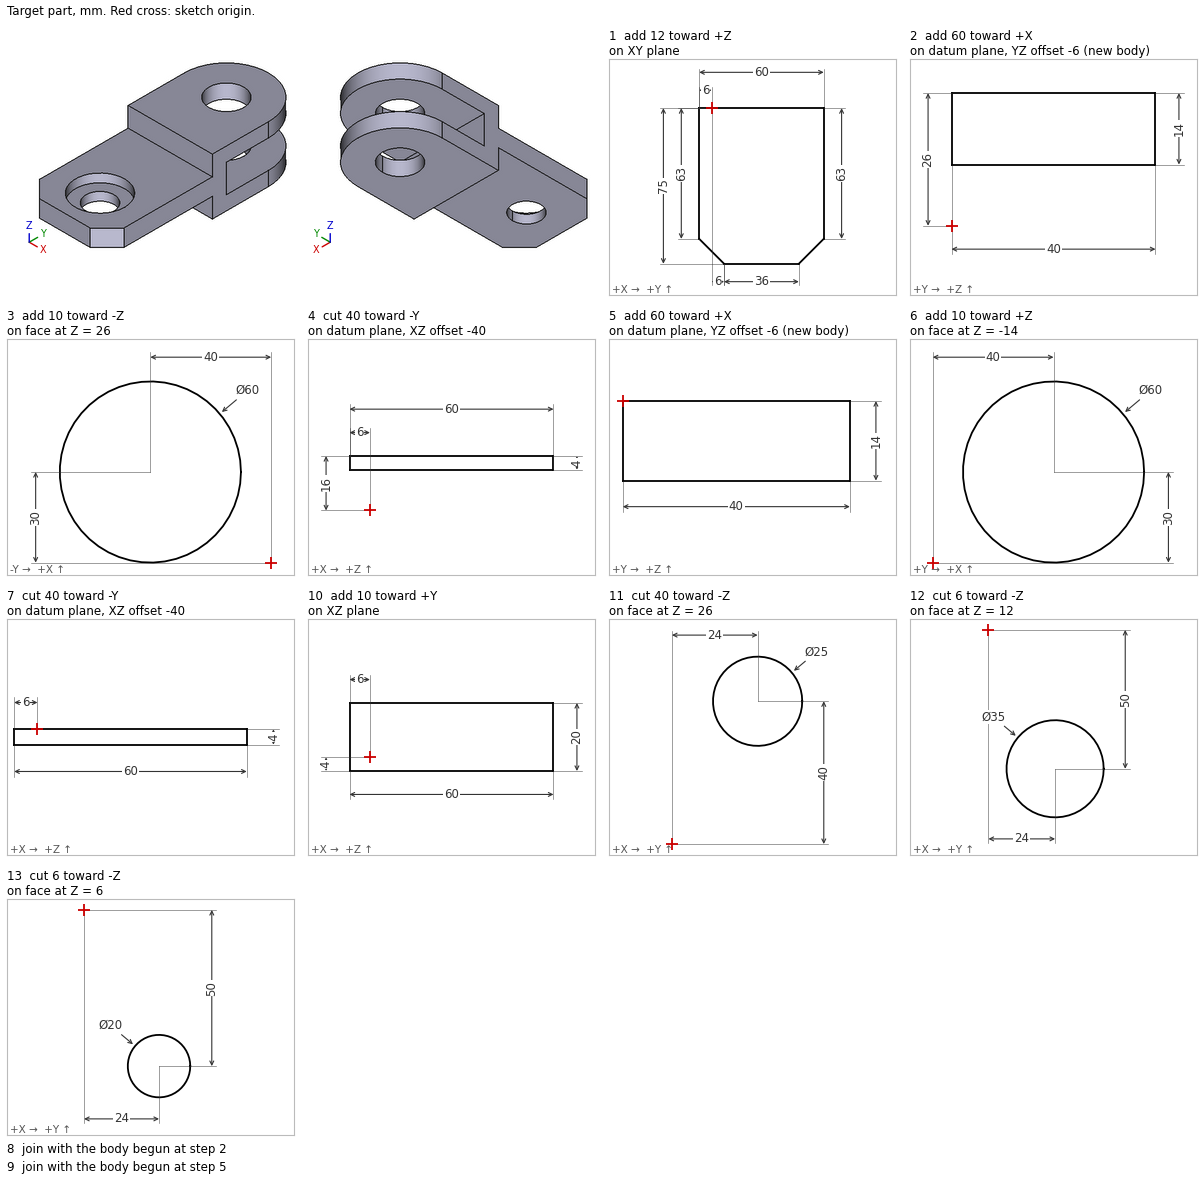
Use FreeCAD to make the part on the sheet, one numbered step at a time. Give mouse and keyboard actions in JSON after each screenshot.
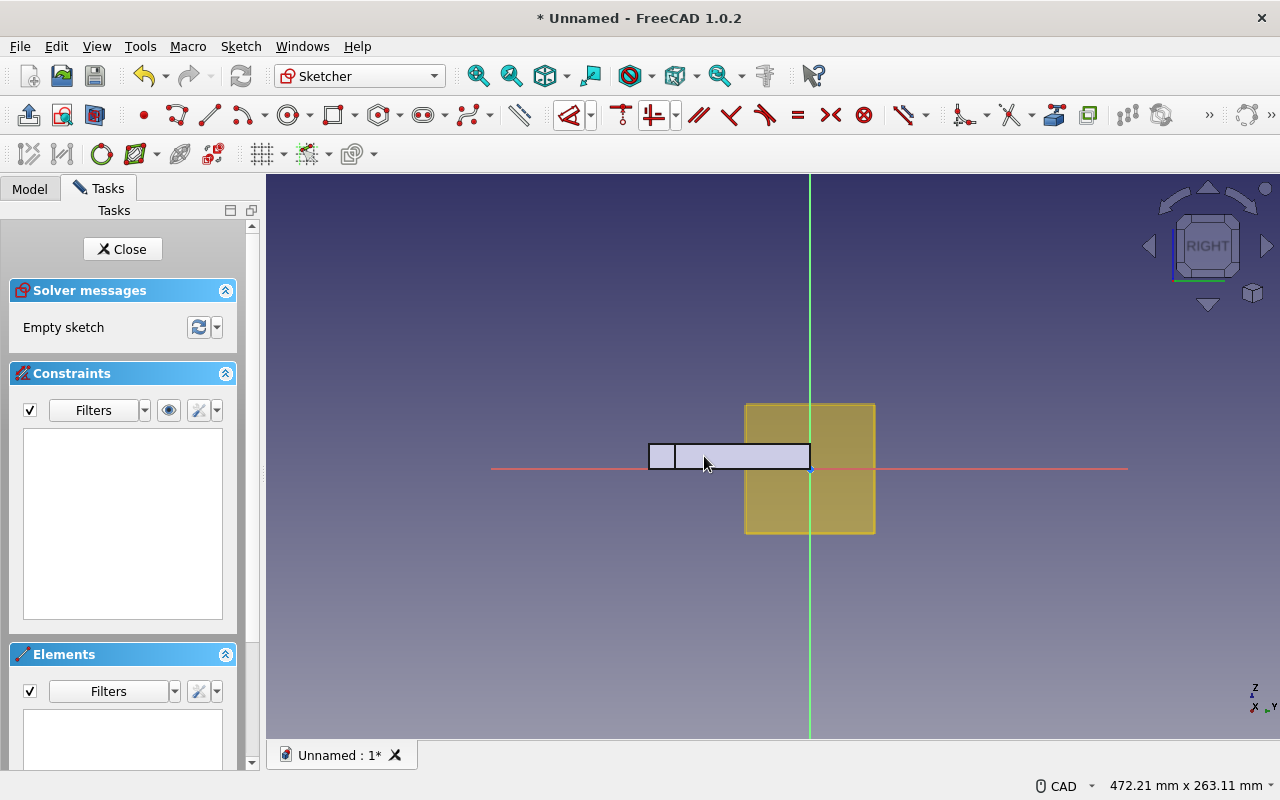
{"action": "scroll", "coordinate": [883, 438], "scroll_direction": "up", "scroll_amount": 9}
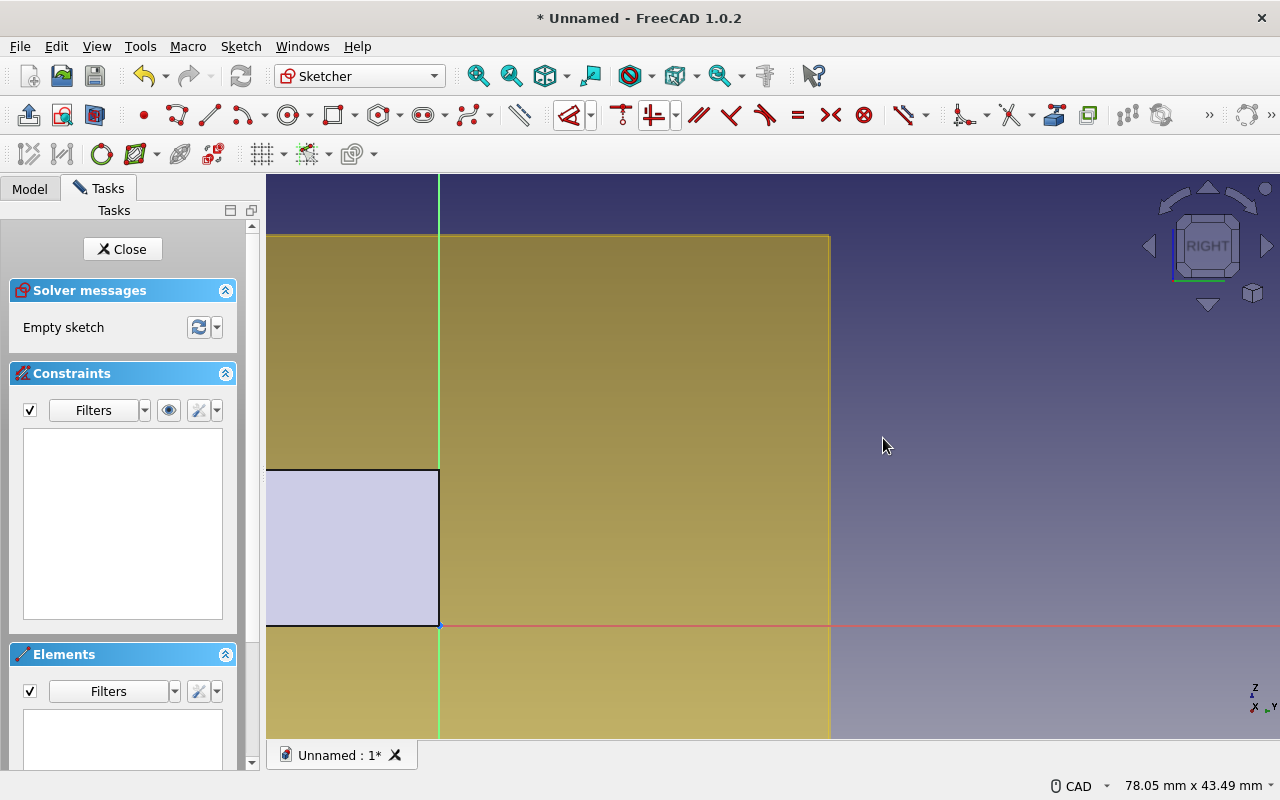
{"action": "left_click", "coordinate": [332, 116]}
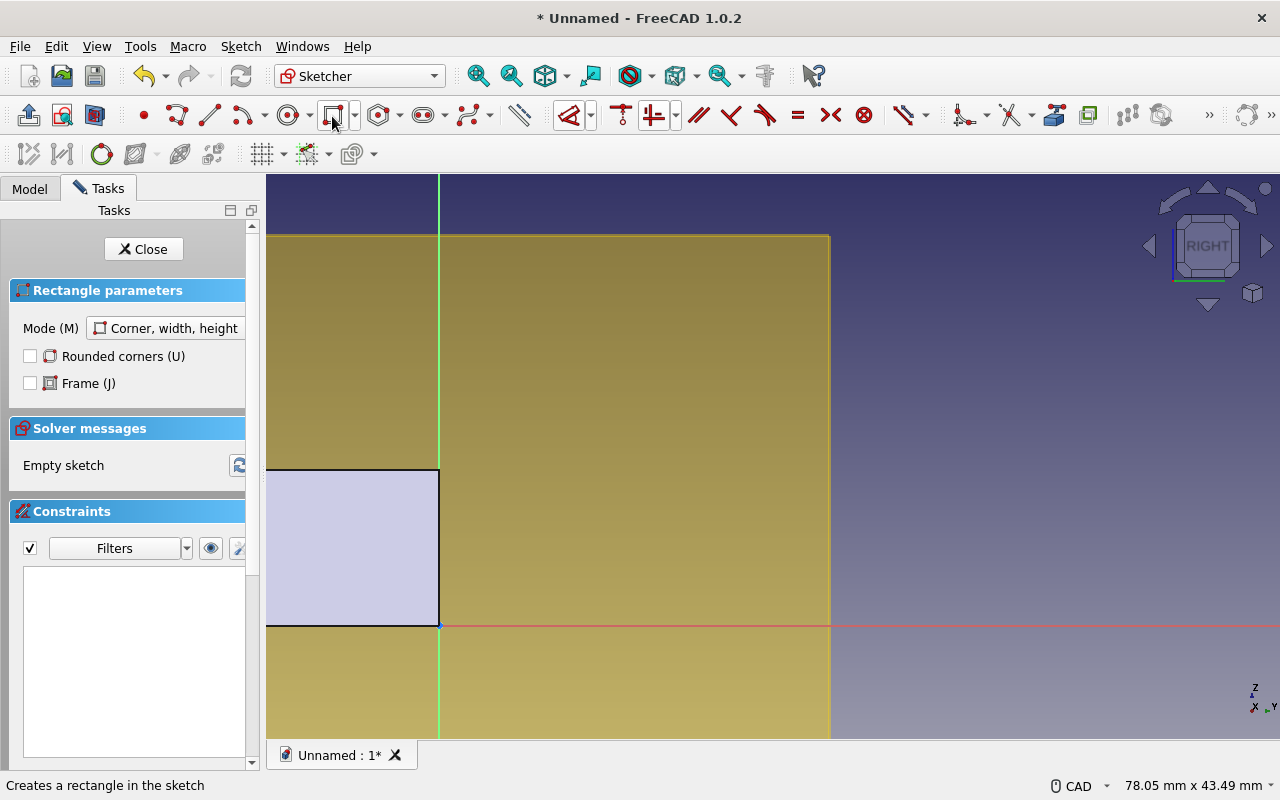
{"action": "left_click", "coordinate": [439, 288]}
{"action": "mouse_move", "coordinate": [959, 470]}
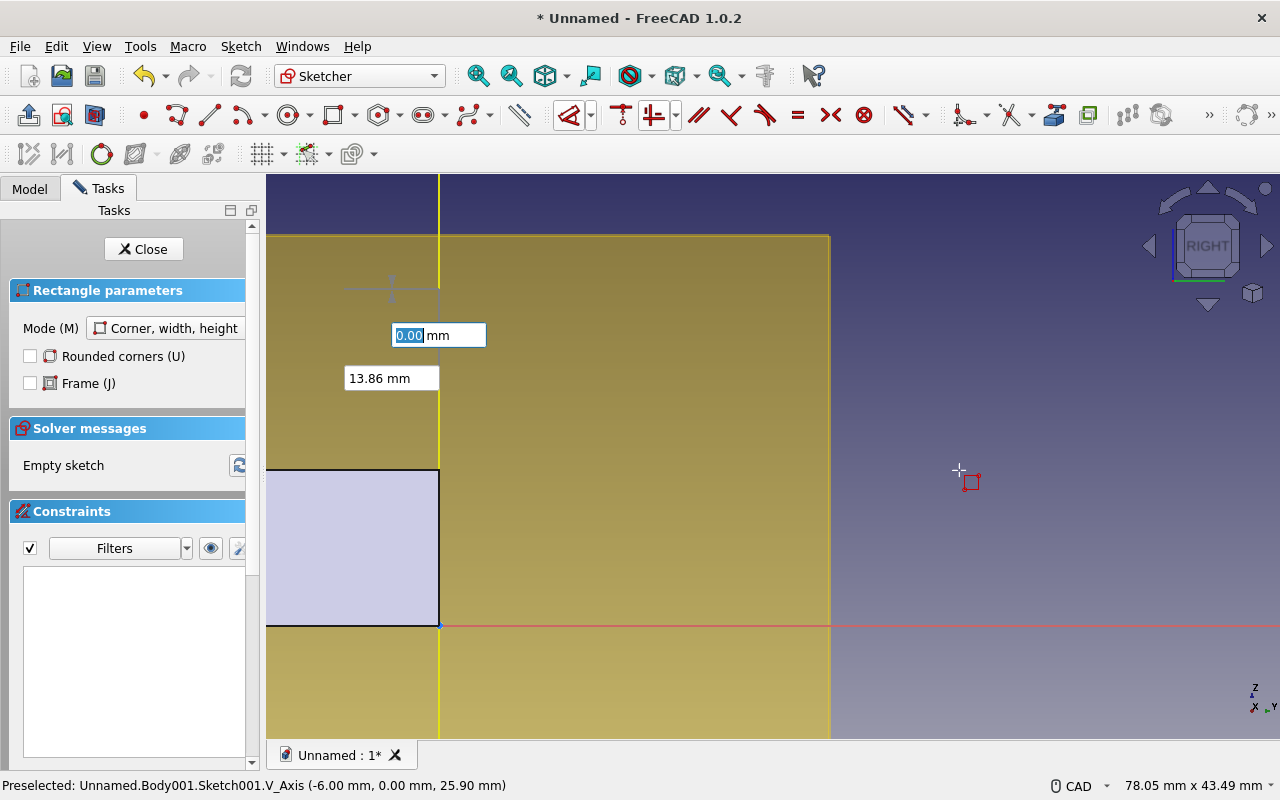
{"action": "type", "text": "40"}
{"action": "key", "text": "Tab"}
{"action": "type", "text": "14"}
{"action": "key", "text": "Return"}
{"action": "key", "text": "Escape"}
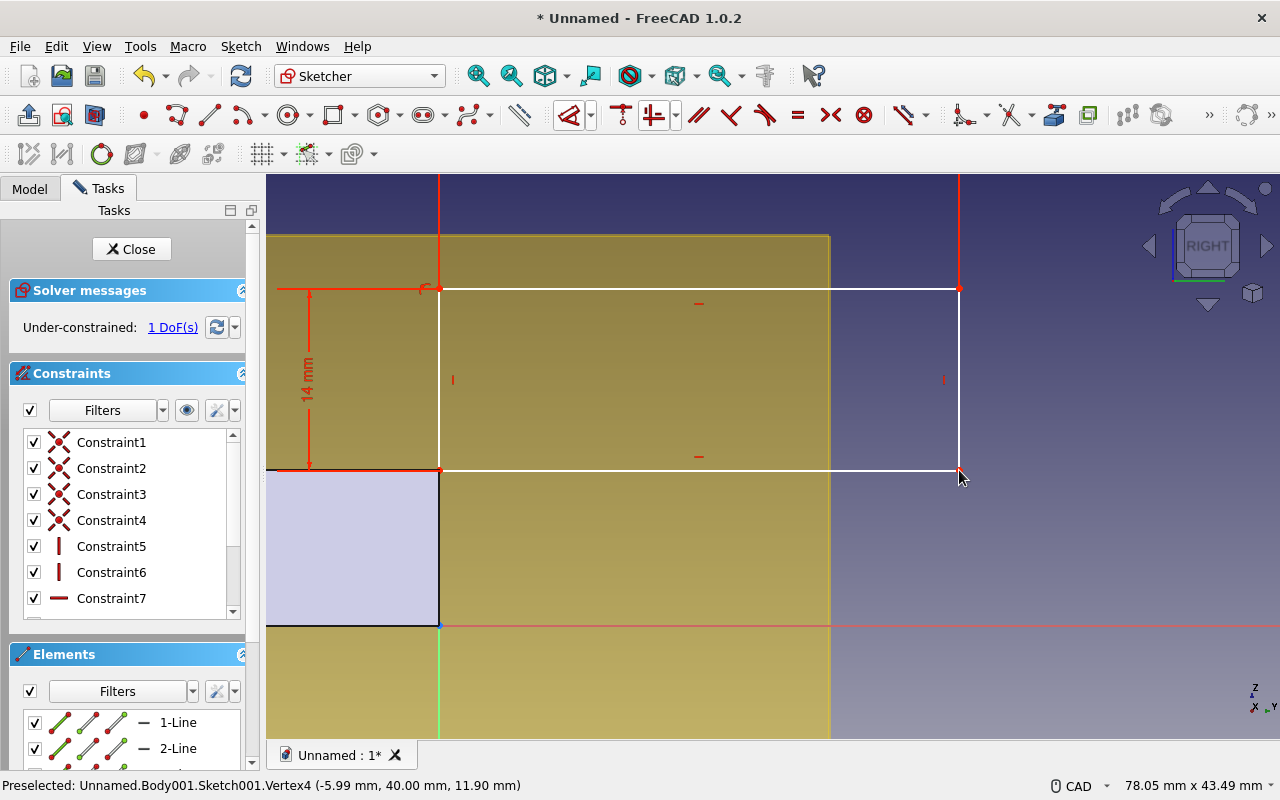
{"action": "left_click", "coordinate": [439, 289]}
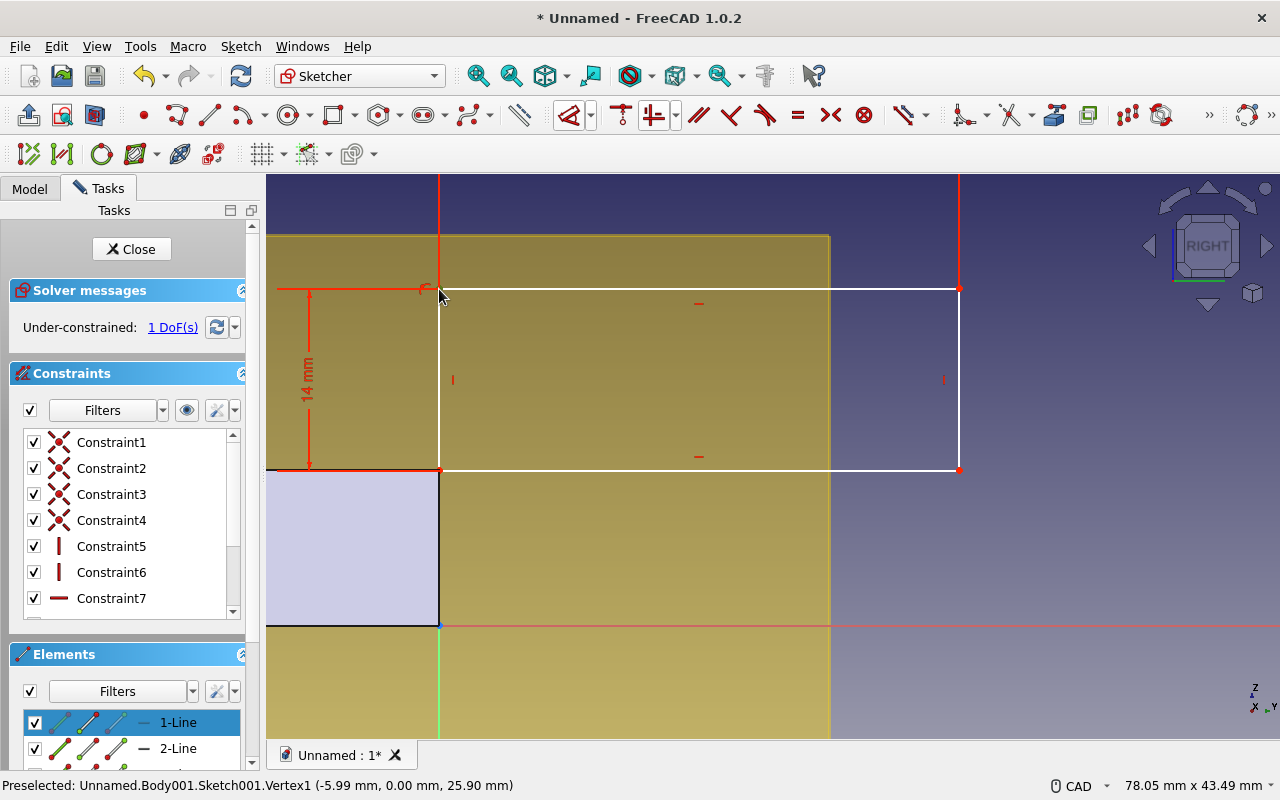
{"action": "left_click", "coordinate": [590, 116]}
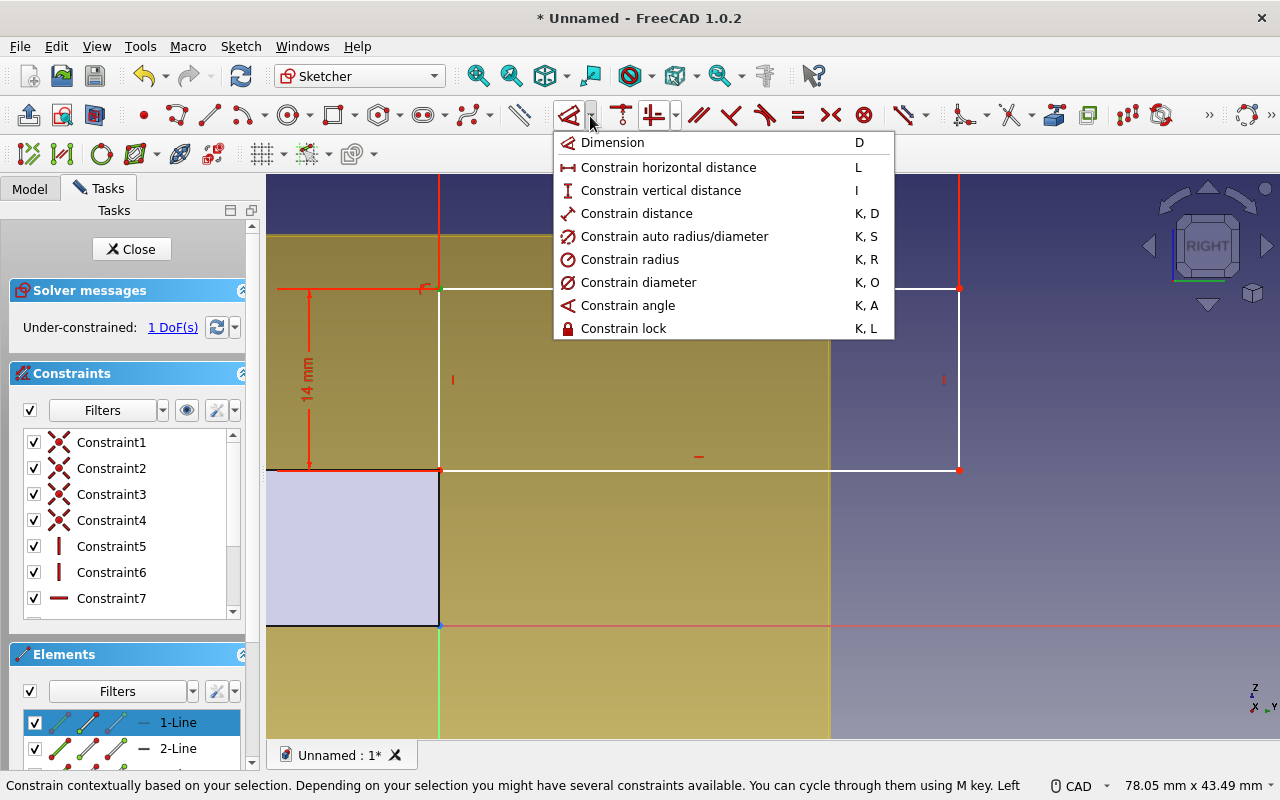
{"action": "left_click", "coordinate": [724, 190]}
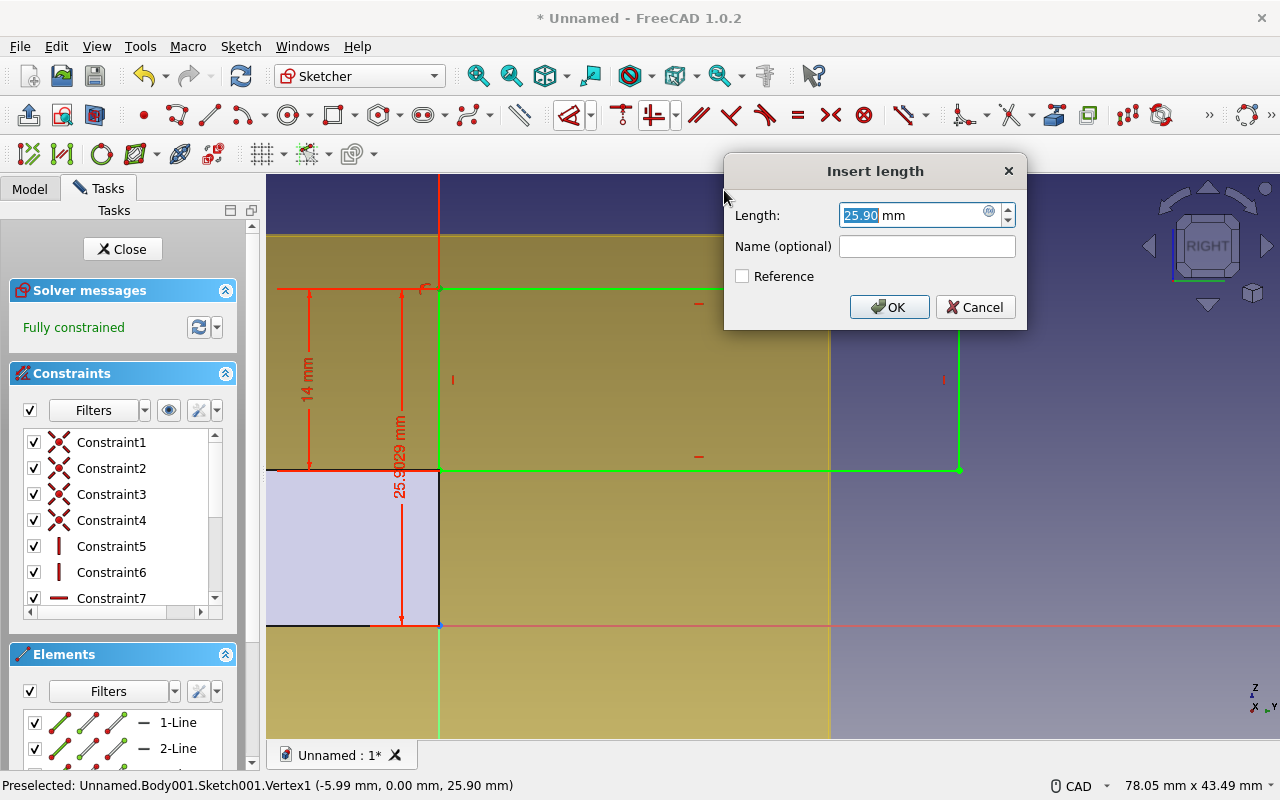
{"action": "type", "text": "26"}
{"action": "key", "text": "Return"}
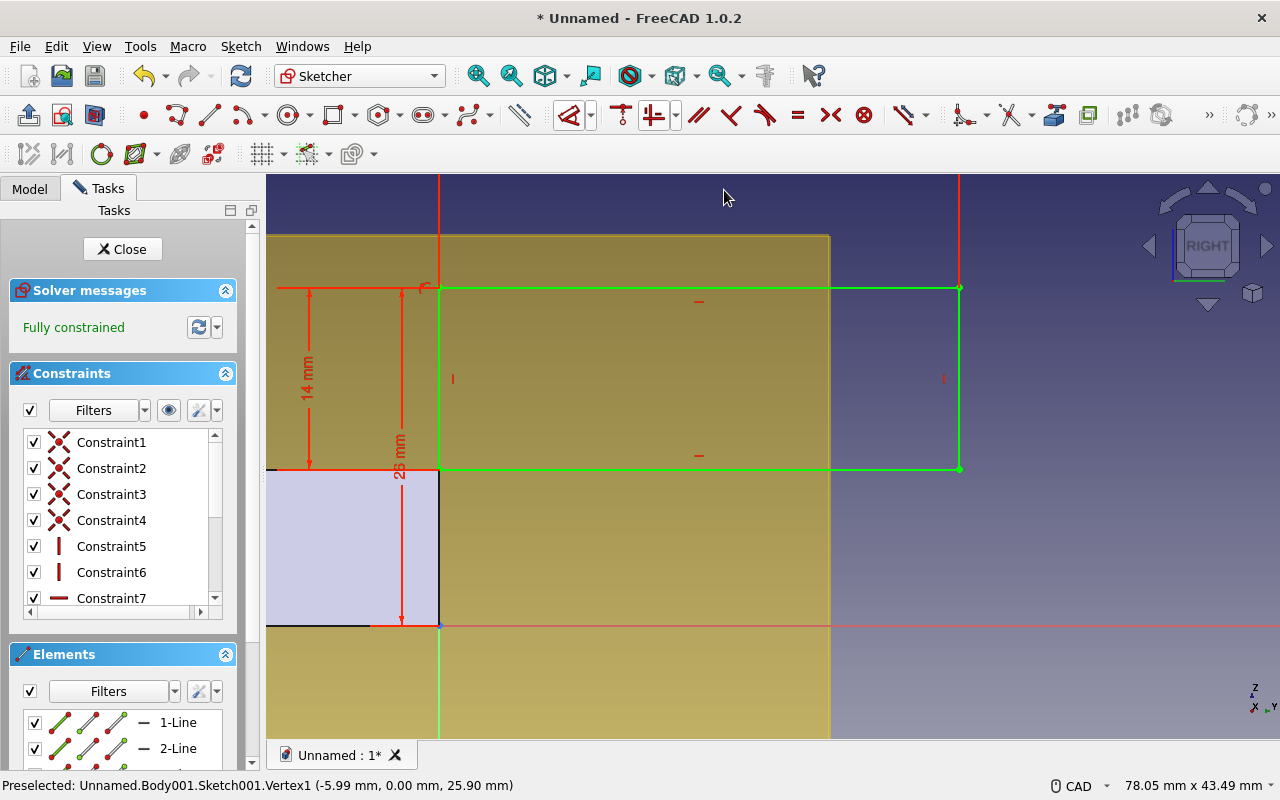
{"action": "left_click", "coordinate": [123, 249]}